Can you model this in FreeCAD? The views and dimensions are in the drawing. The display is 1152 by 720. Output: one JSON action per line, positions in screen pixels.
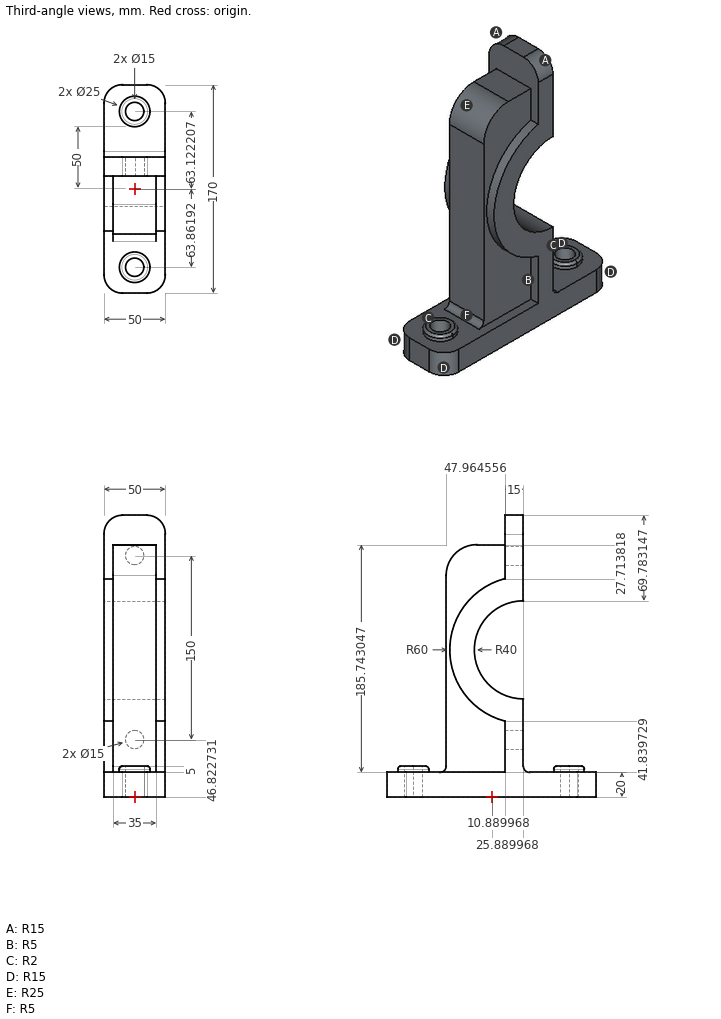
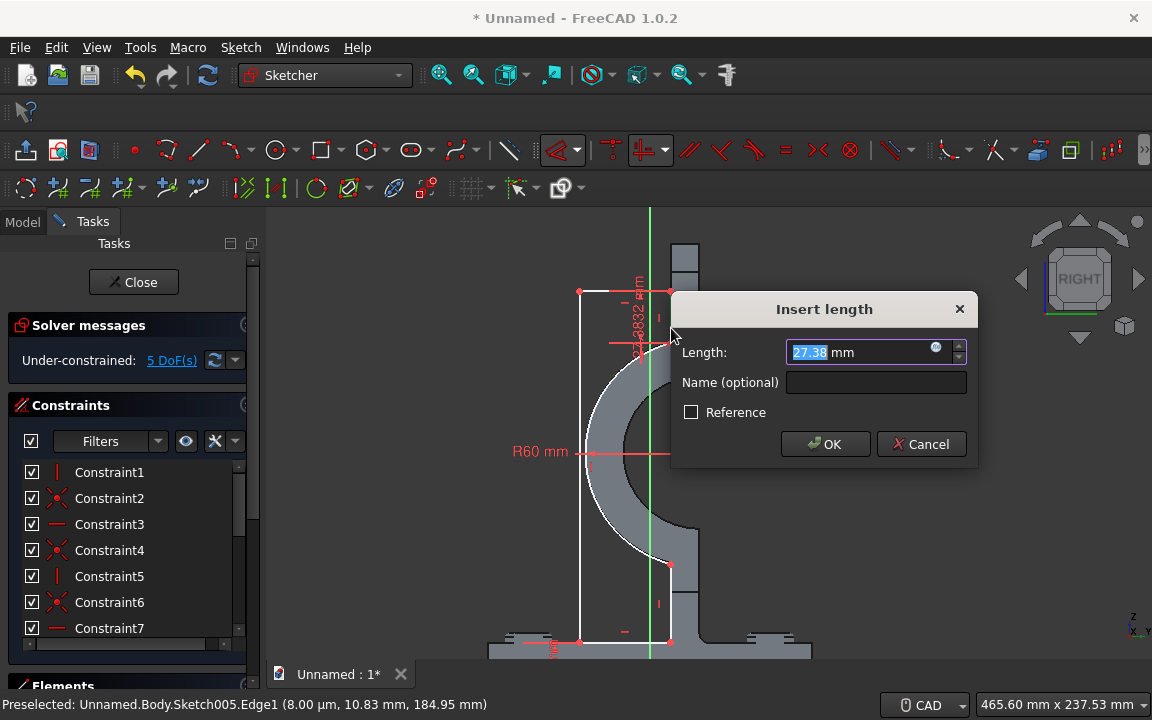
{"action": "type", "text": "27.713818"}
{"action": "key", "text": "Return"}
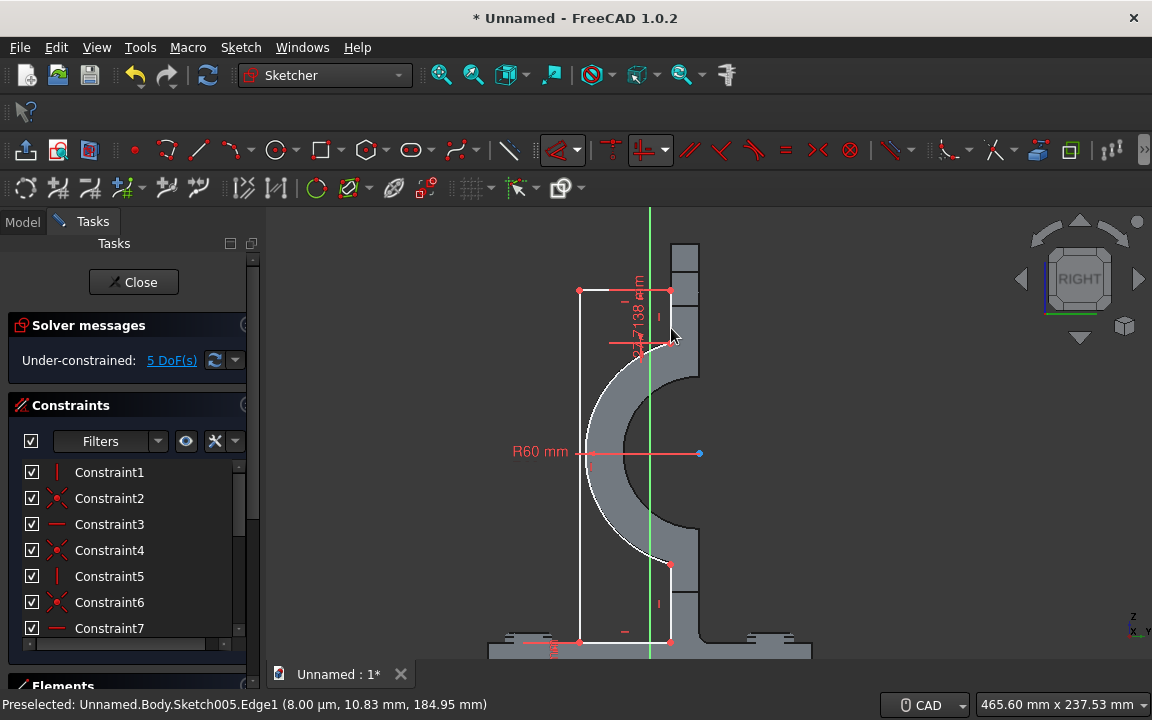
{"action": "left_click", "coordinate": [607, 290]}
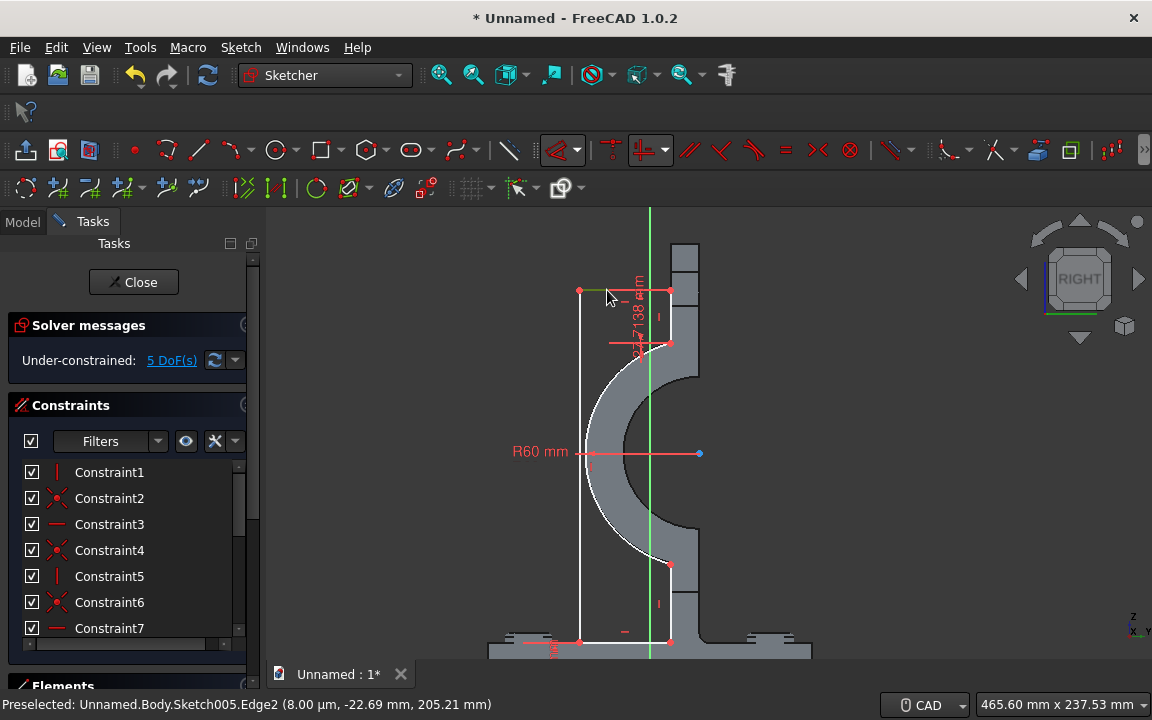
{"action": "key", "text": "l"}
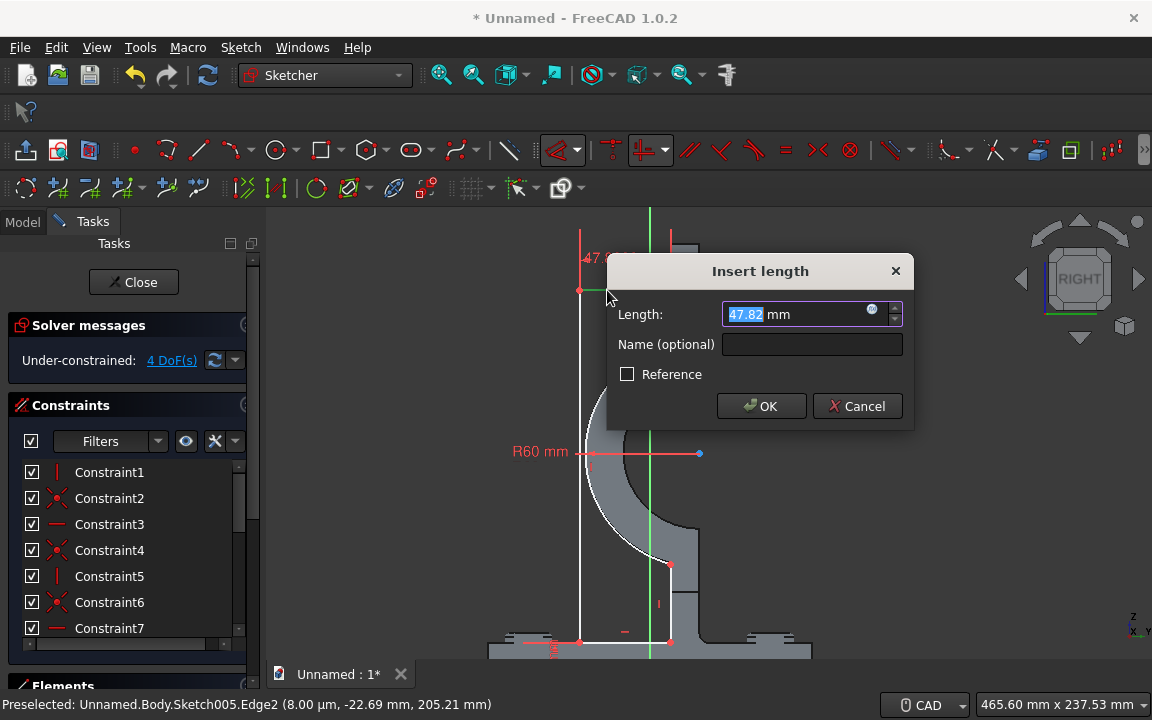
{"action": "type", "text": "47.964556"}
{"action": "key", "text": "Return"}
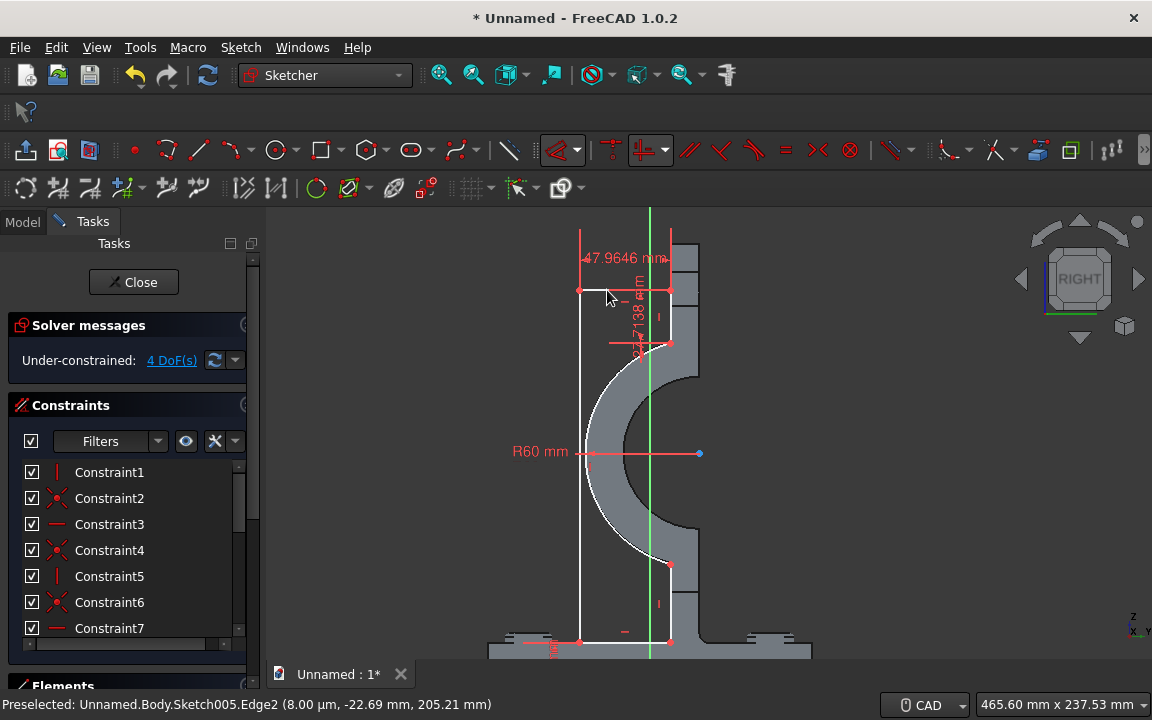
{"action": "scroll", "coordinate": [671, 327], "scroll_direction": "down", "scroll_amount": 2}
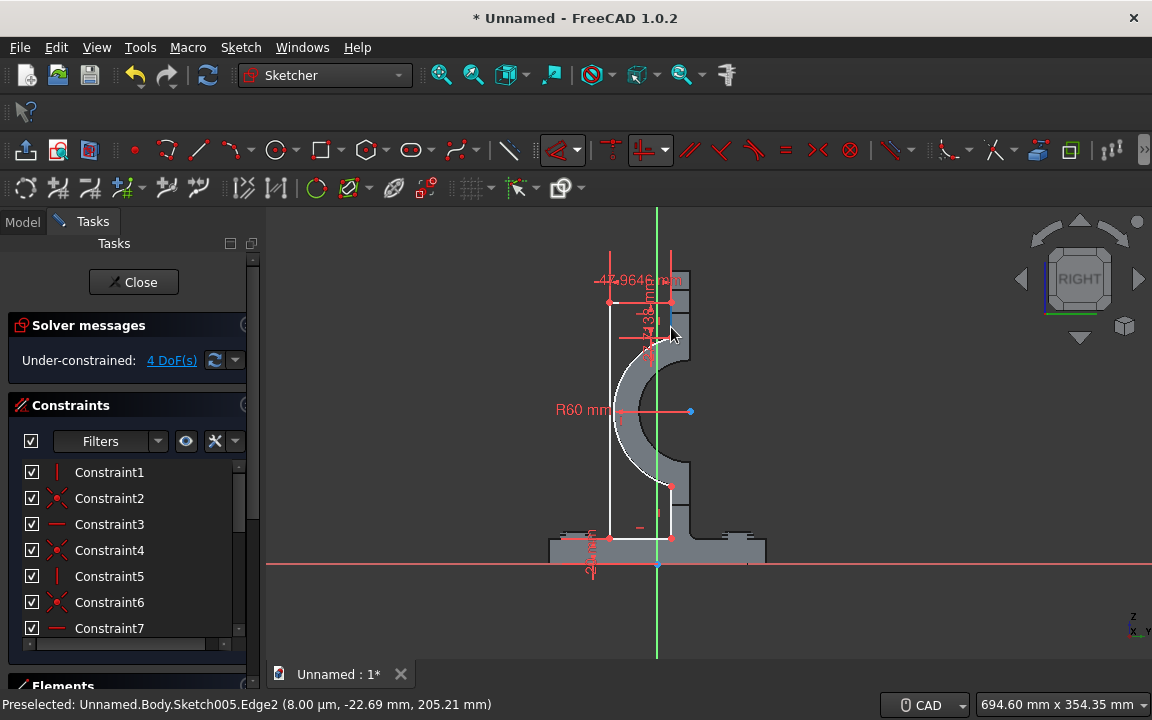
{"action": "left_click", "coordinate": [628, 539]}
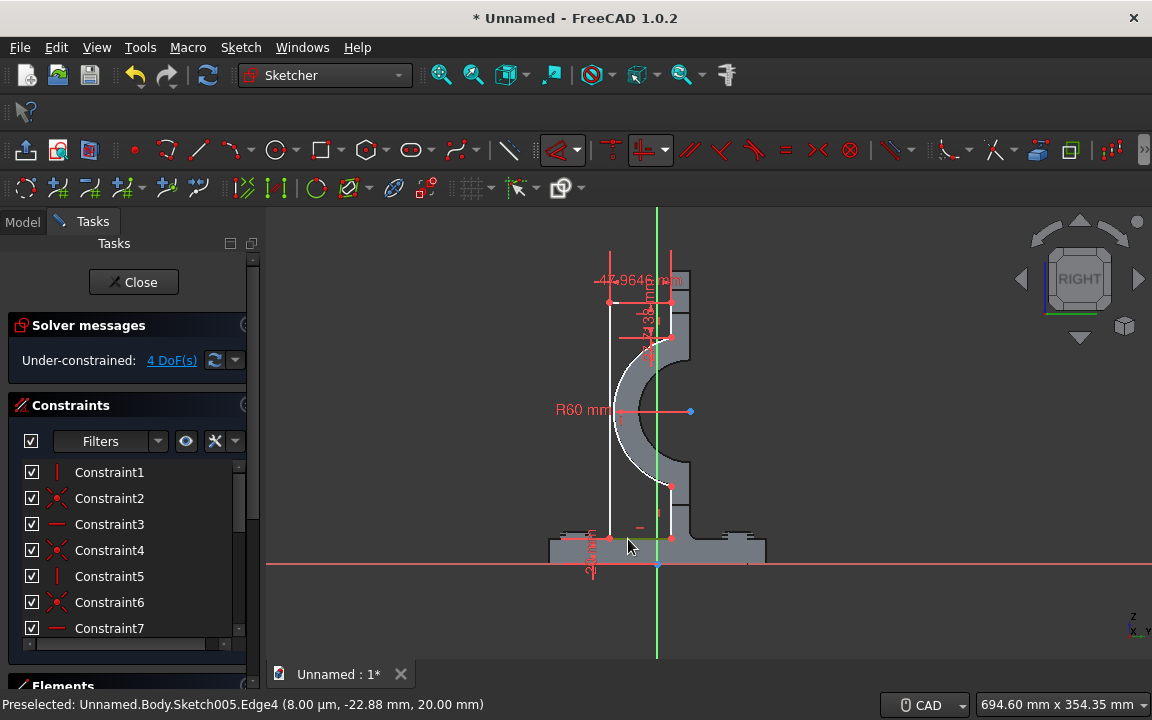
{"action": "key", "text": "l"}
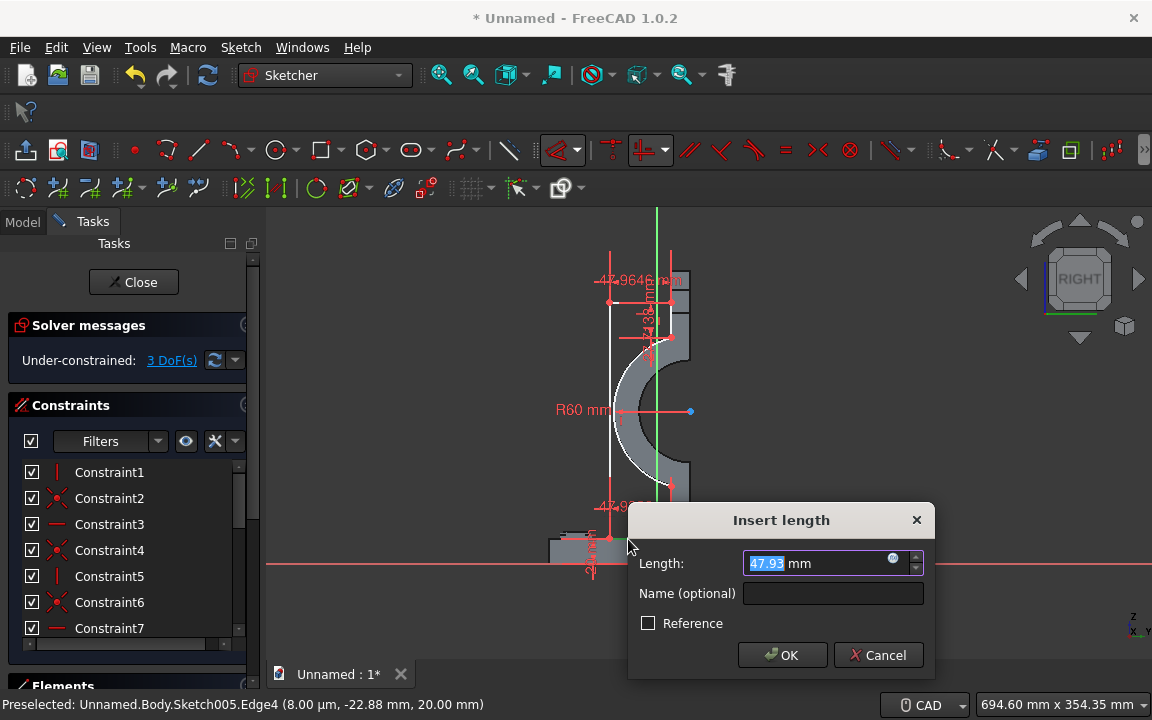
{"action": "type", "text": "47.964556"}
{"action": "key", "text": "Return"}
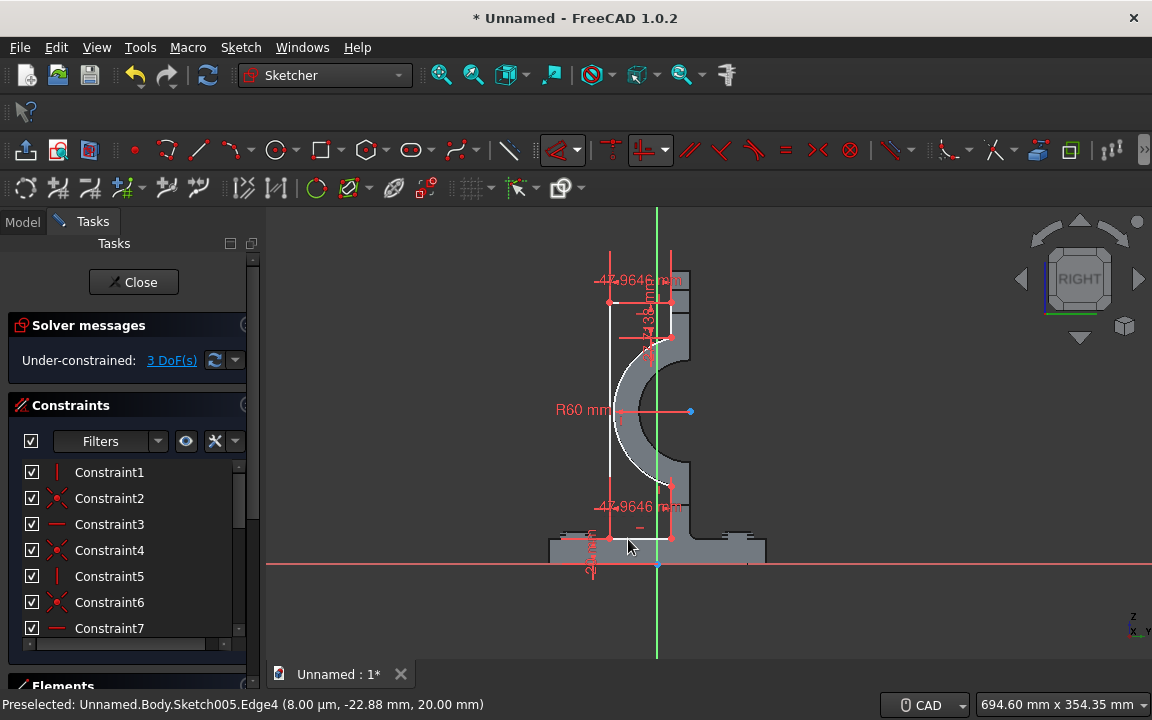
{"action": "left_click", "coordinate": [671, 523]}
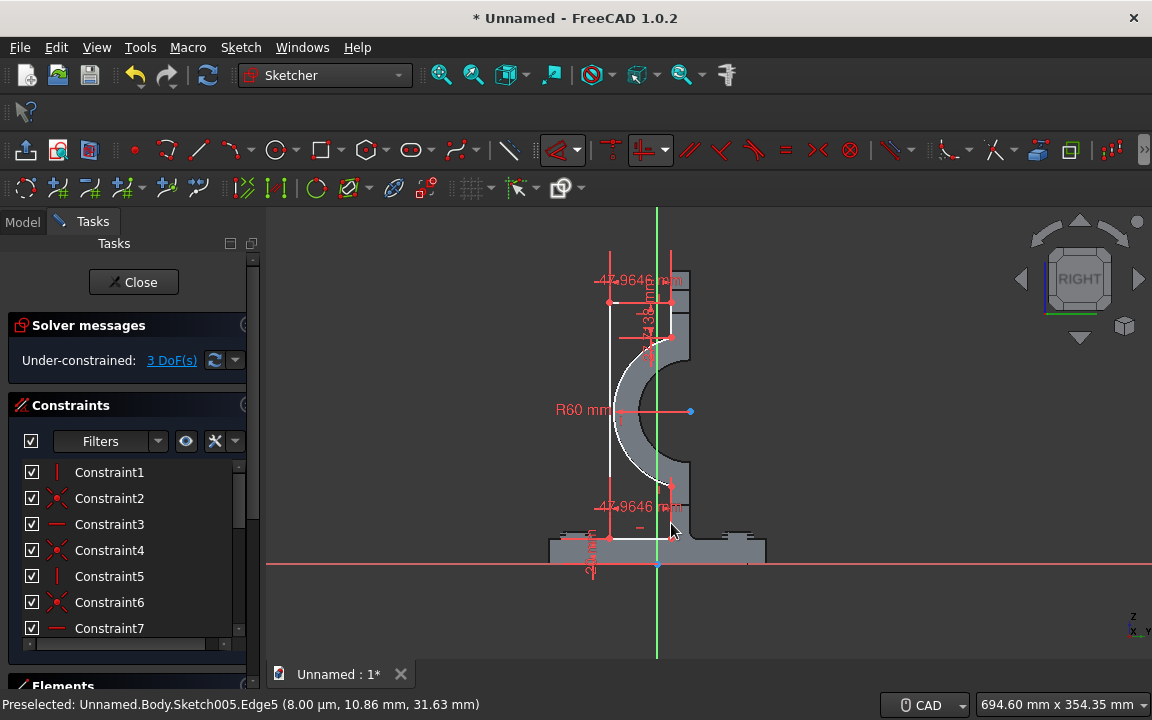
{"action": "key", "text": "i"}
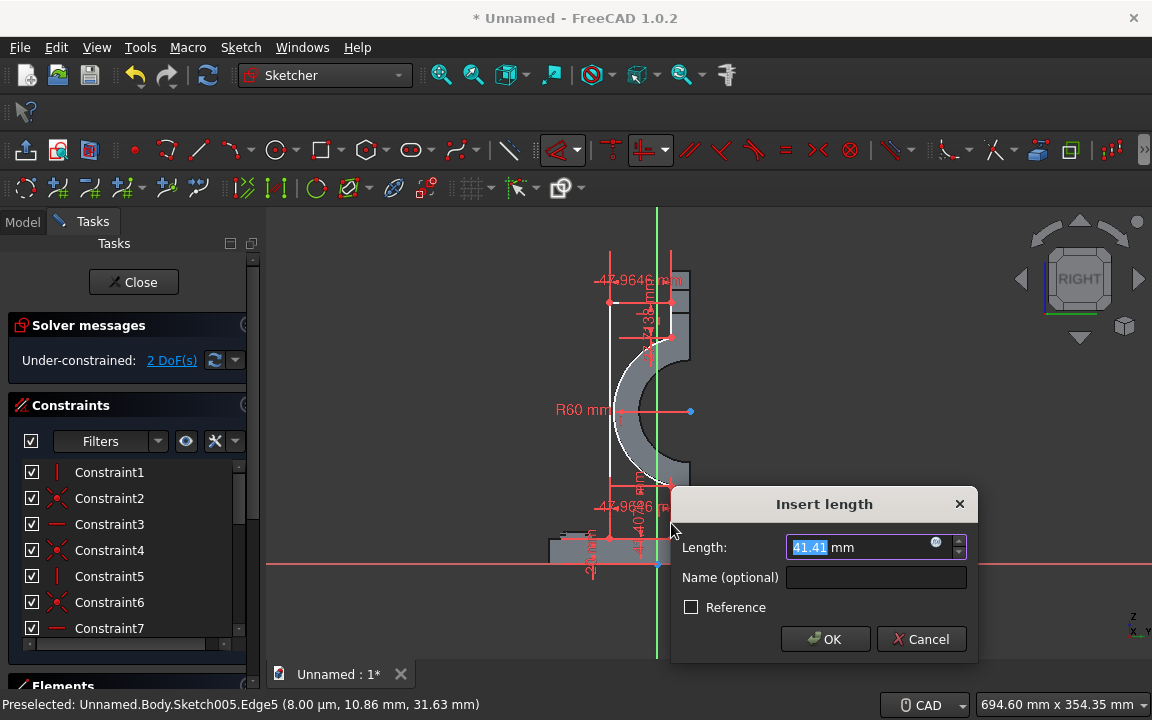
{"action": "type", "text": "41.839729"}
{"action": "key", "text": "Return"}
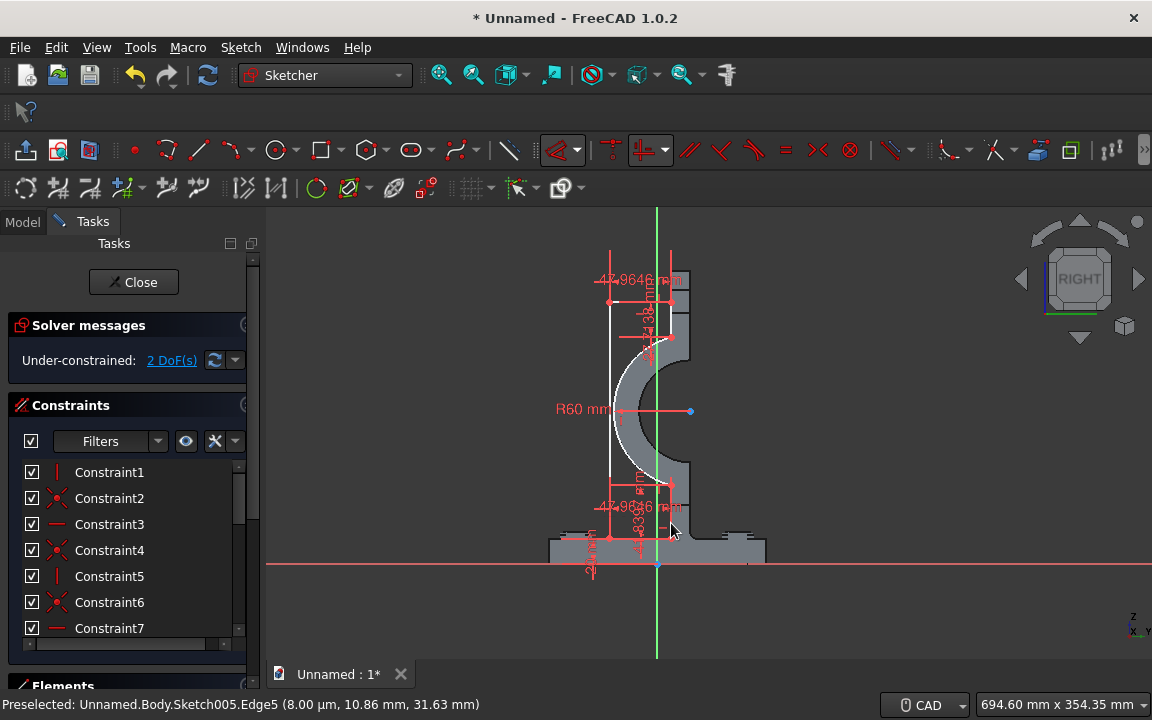
{"action": "left_click", "coordinate": [610, 373]}